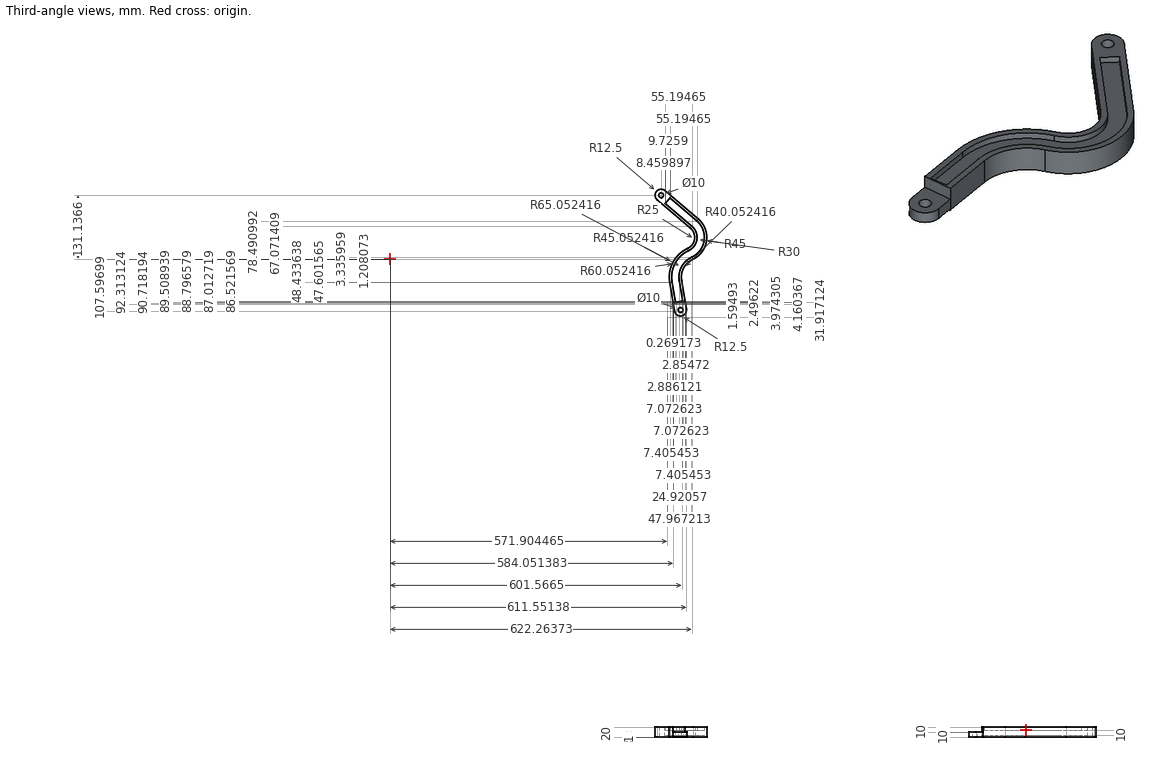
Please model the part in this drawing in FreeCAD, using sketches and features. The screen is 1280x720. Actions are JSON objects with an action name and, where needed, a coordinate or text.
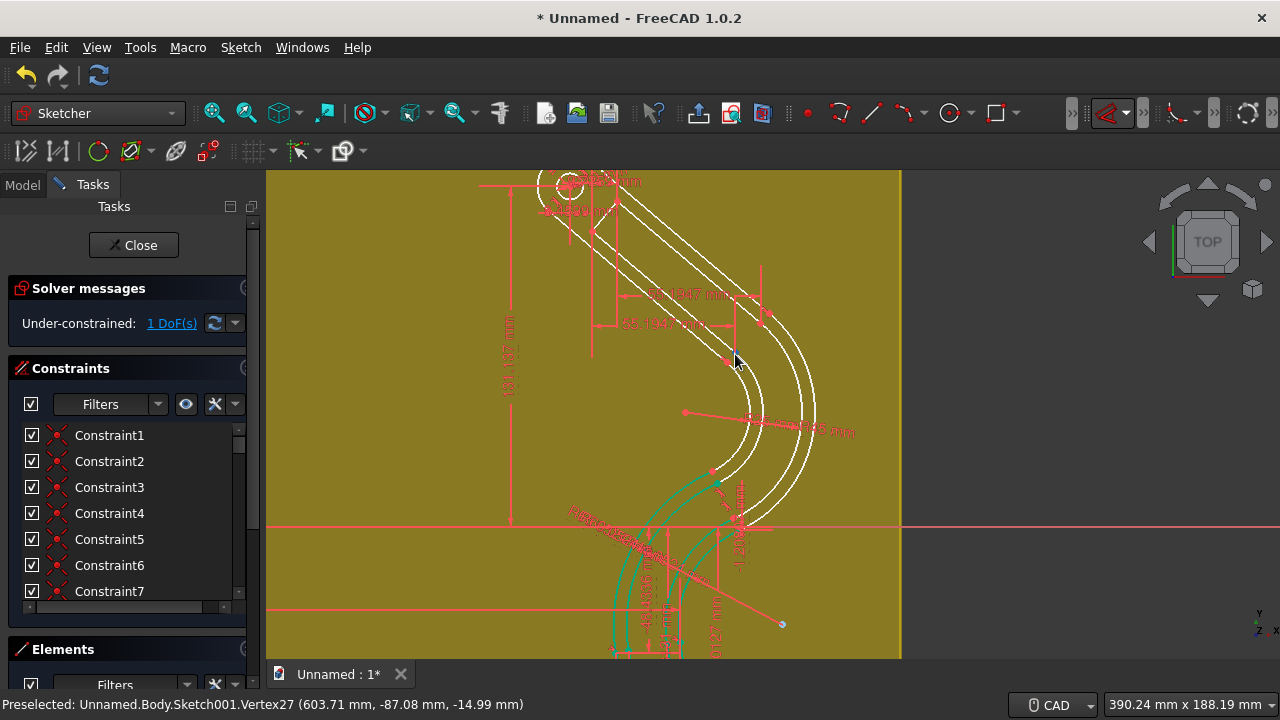
{"action": "left_click", "coordinate": [735, 353]}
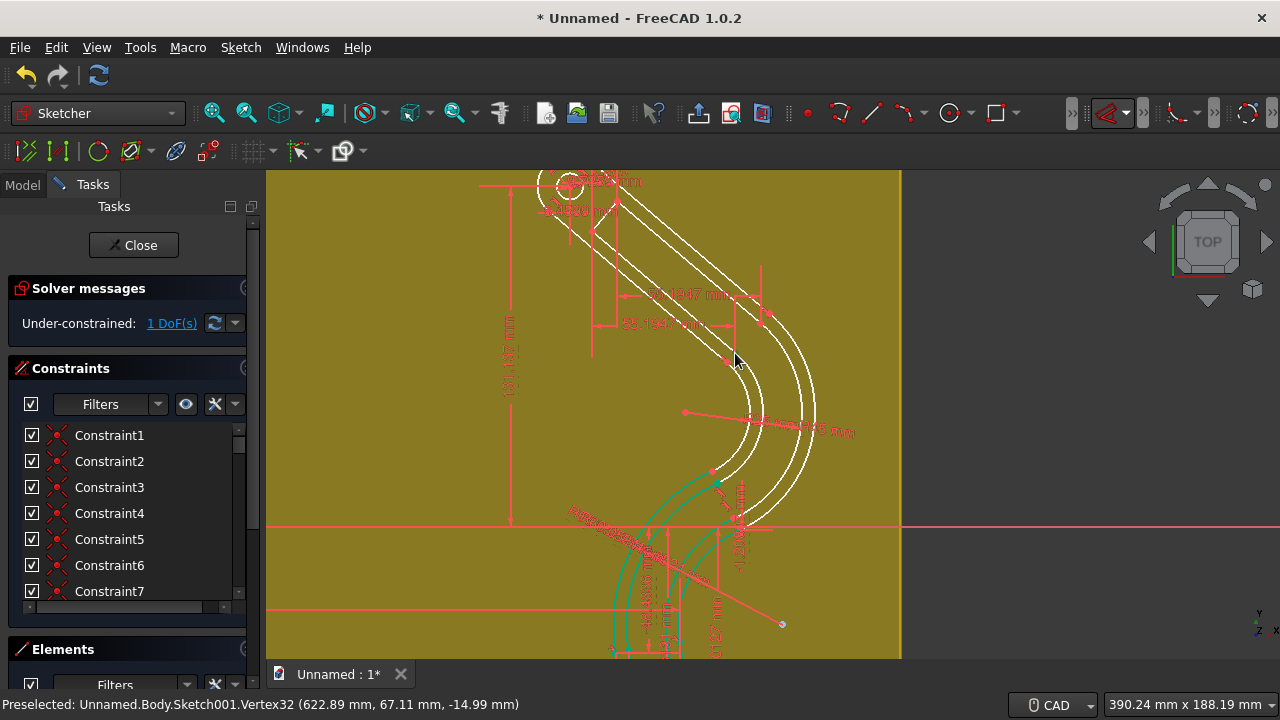
{"action": "key", "text": "i"}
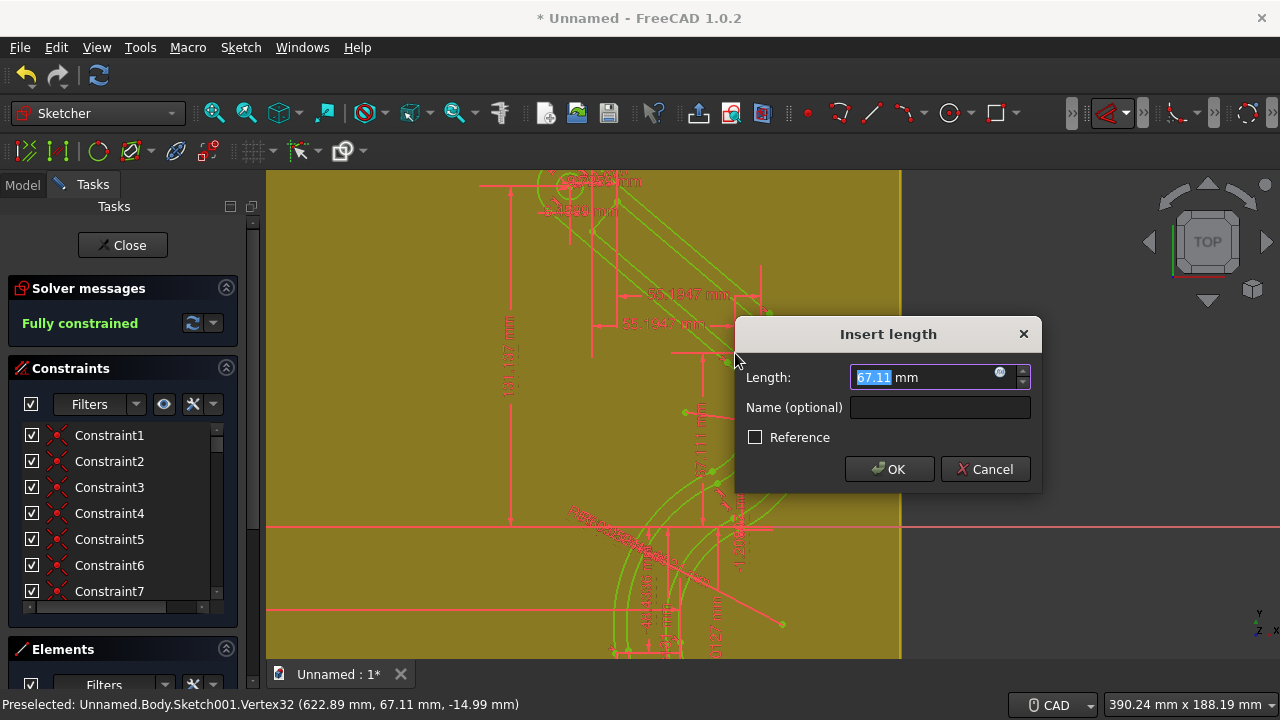
{"action": "type", "text": "67.071409"}
{"action": "key", "text": "Return"}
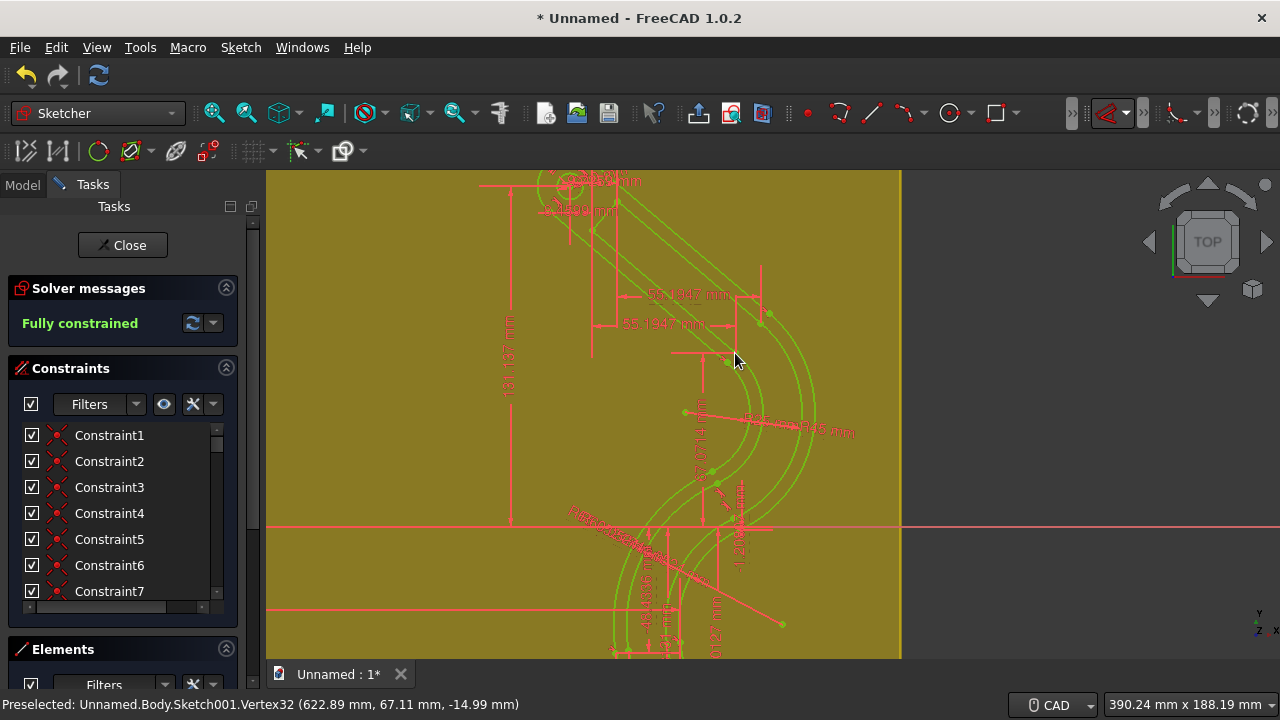
{"action": "left_click", "coordinate": [123, 245]}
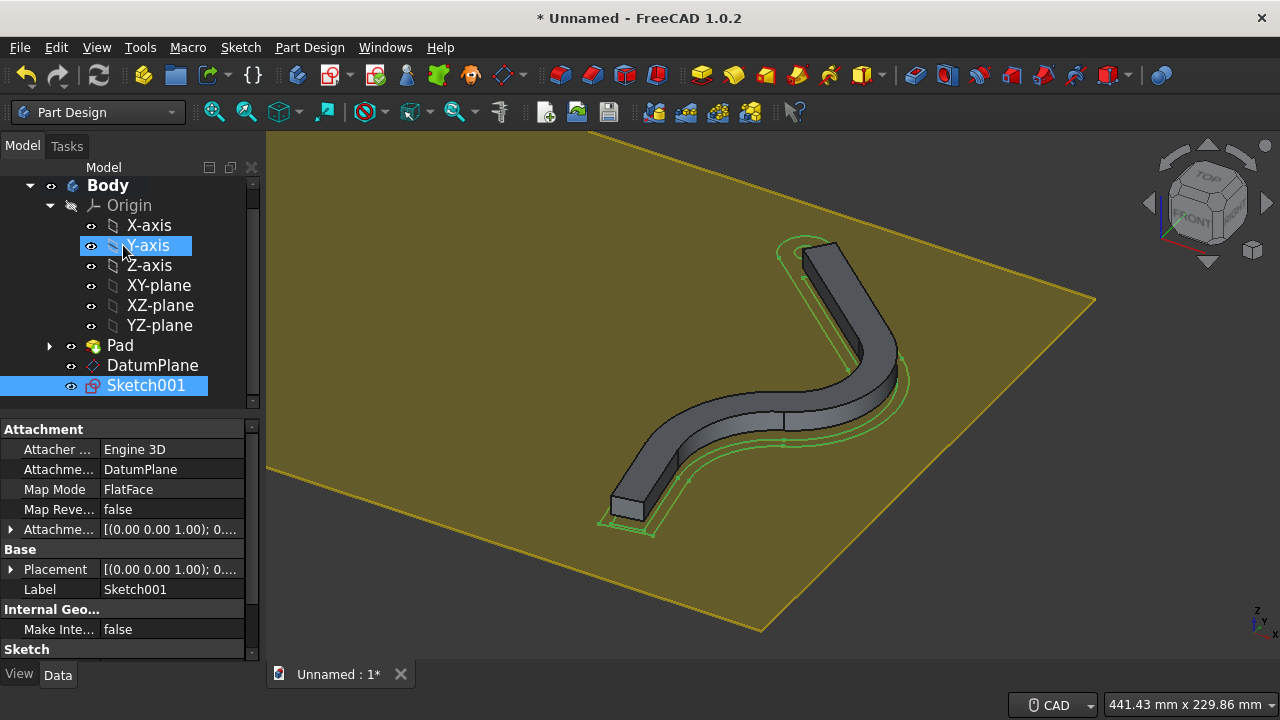
{"action": "left_click", "coordinate": [702, 76]}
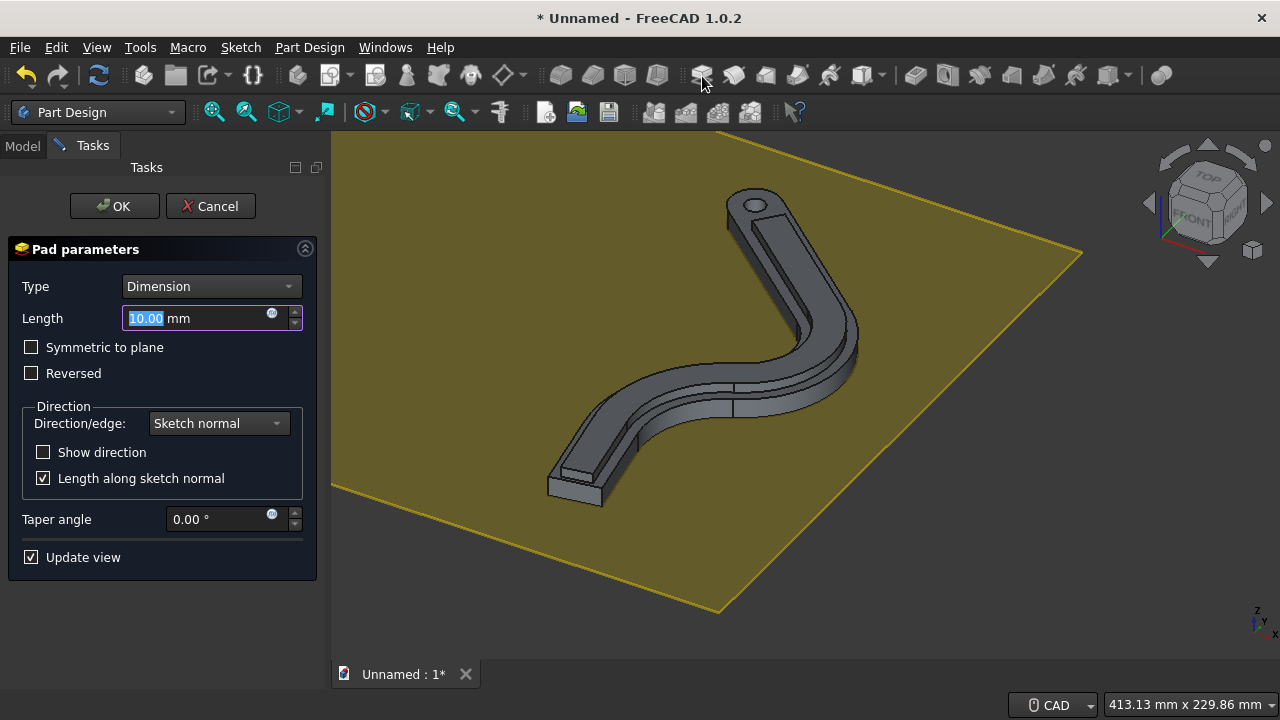
{"action": "type", "text": "20"}
{"action": "key", "text": "Tab"}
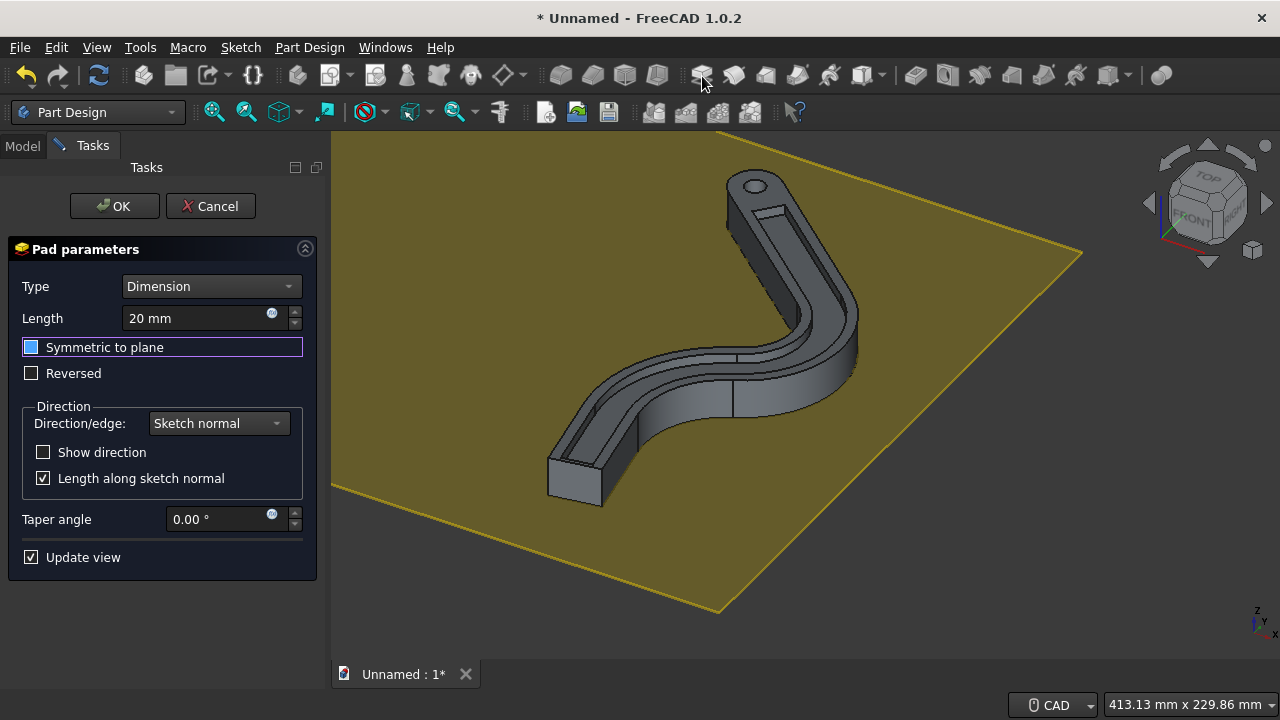
{"action": "left_click", "coordinate": [115, 206]}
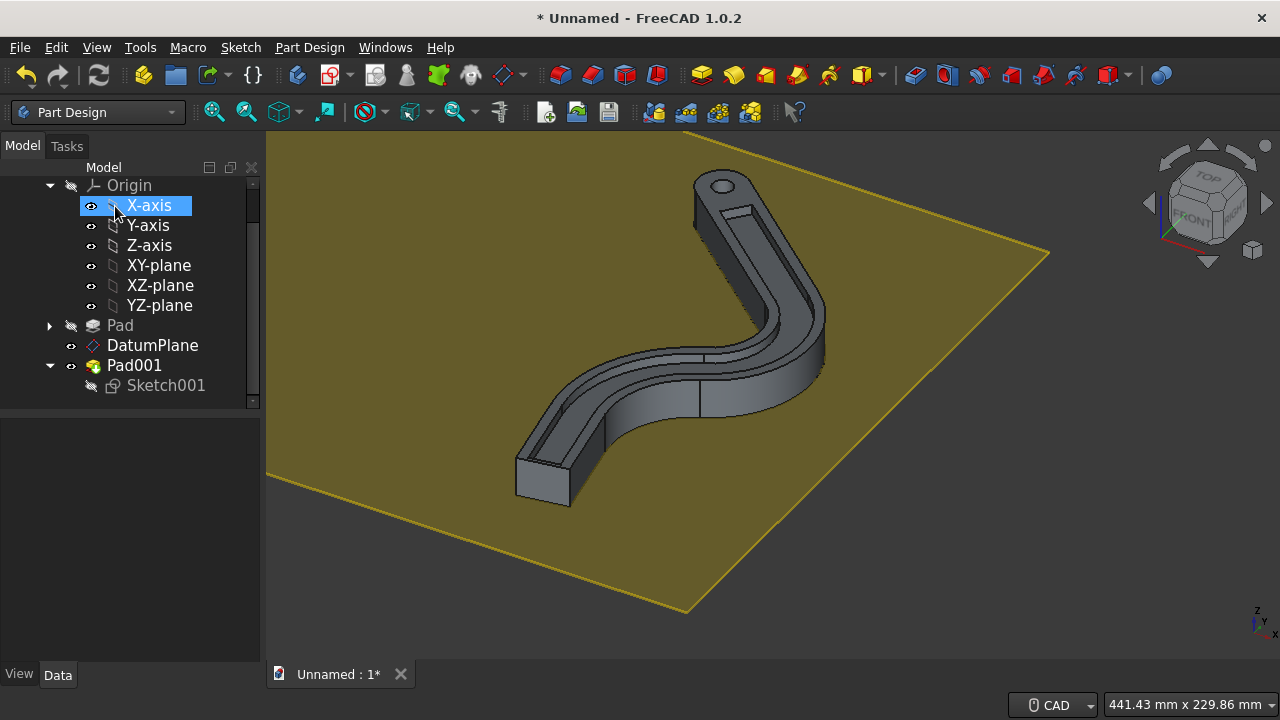
{"action": "left_click", "coordinate": [116, 346]}
{"action": "key", "text": "space"}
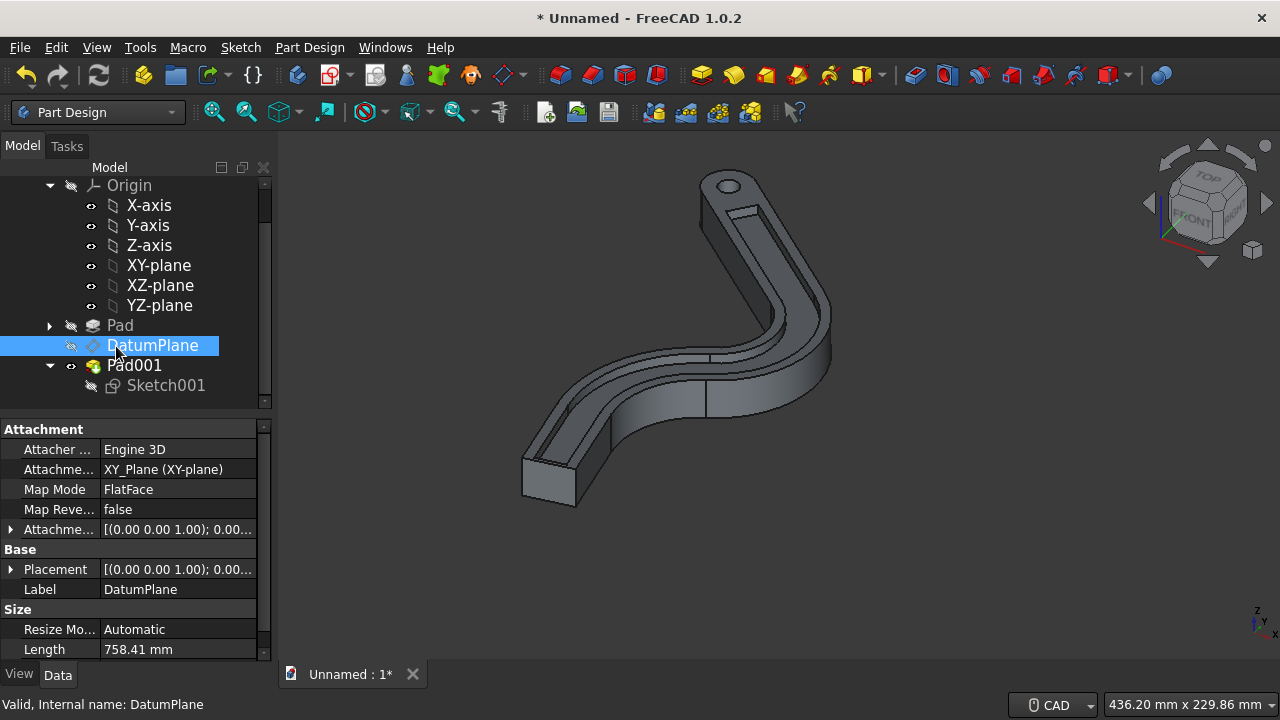
{"action": "left_click", "coordinate": [136, 266]}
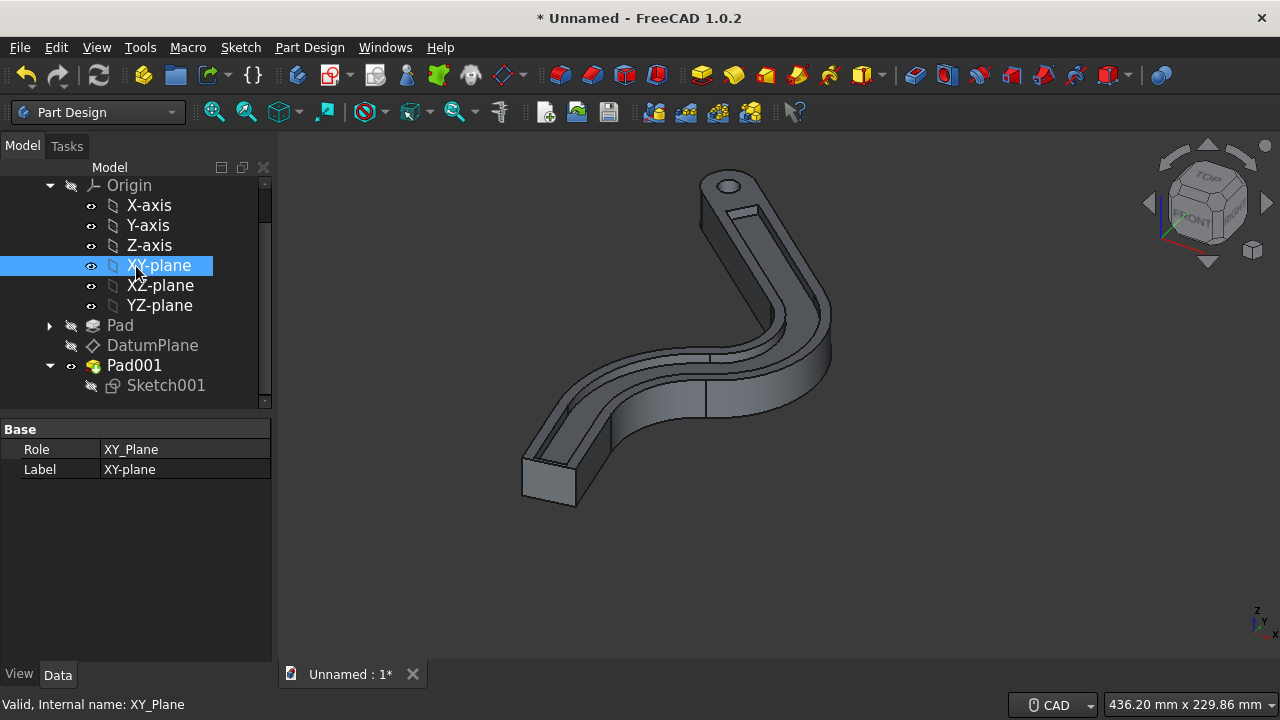
{"action": "left_click", "coordinate": [504, 76]}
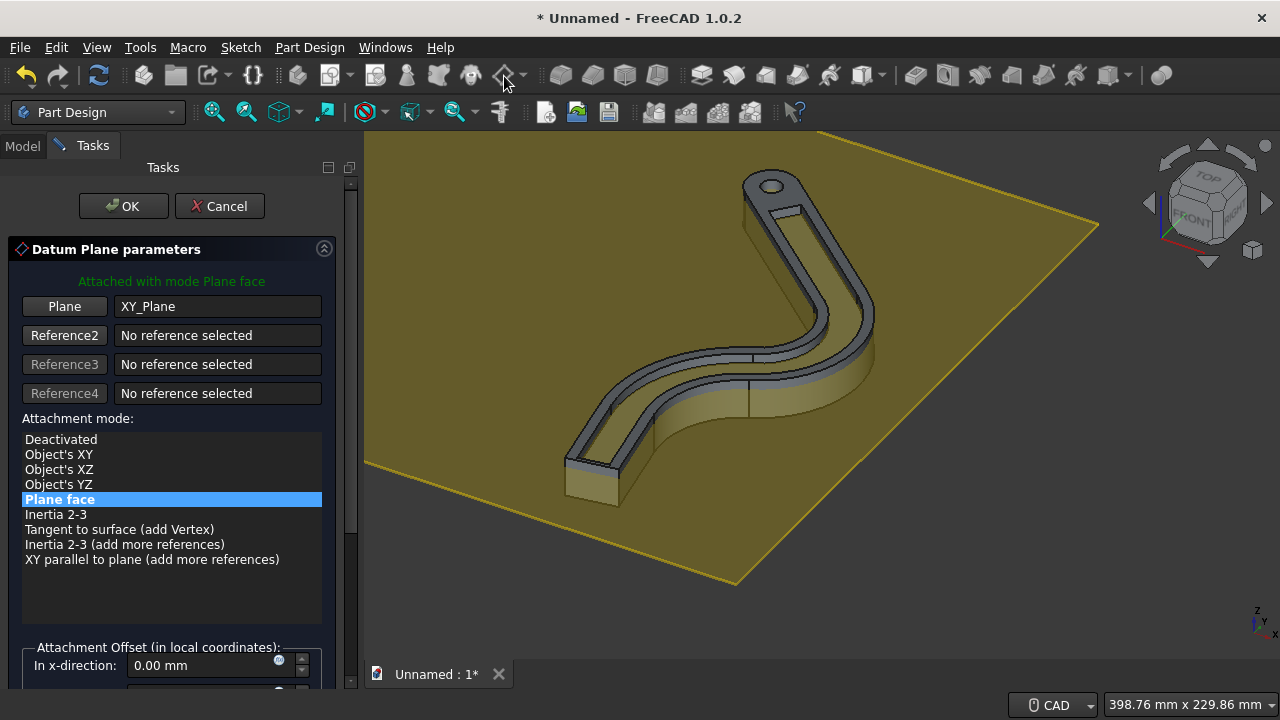
{"action": "scroll", "coordinate": [351, 432], "scroll_direction": "down", "scroll_amount": 2}